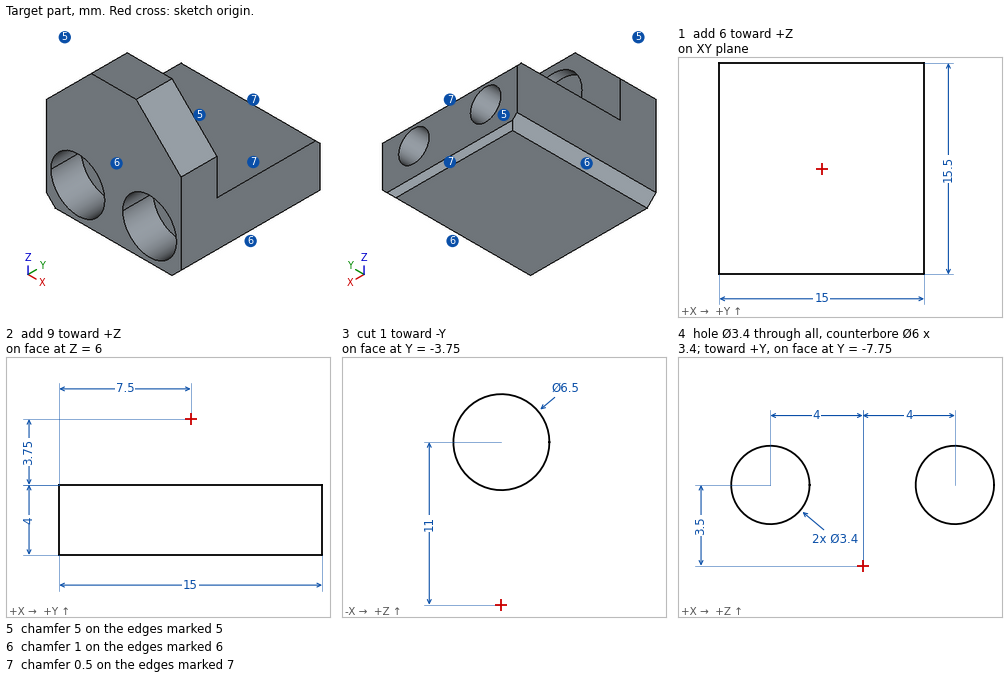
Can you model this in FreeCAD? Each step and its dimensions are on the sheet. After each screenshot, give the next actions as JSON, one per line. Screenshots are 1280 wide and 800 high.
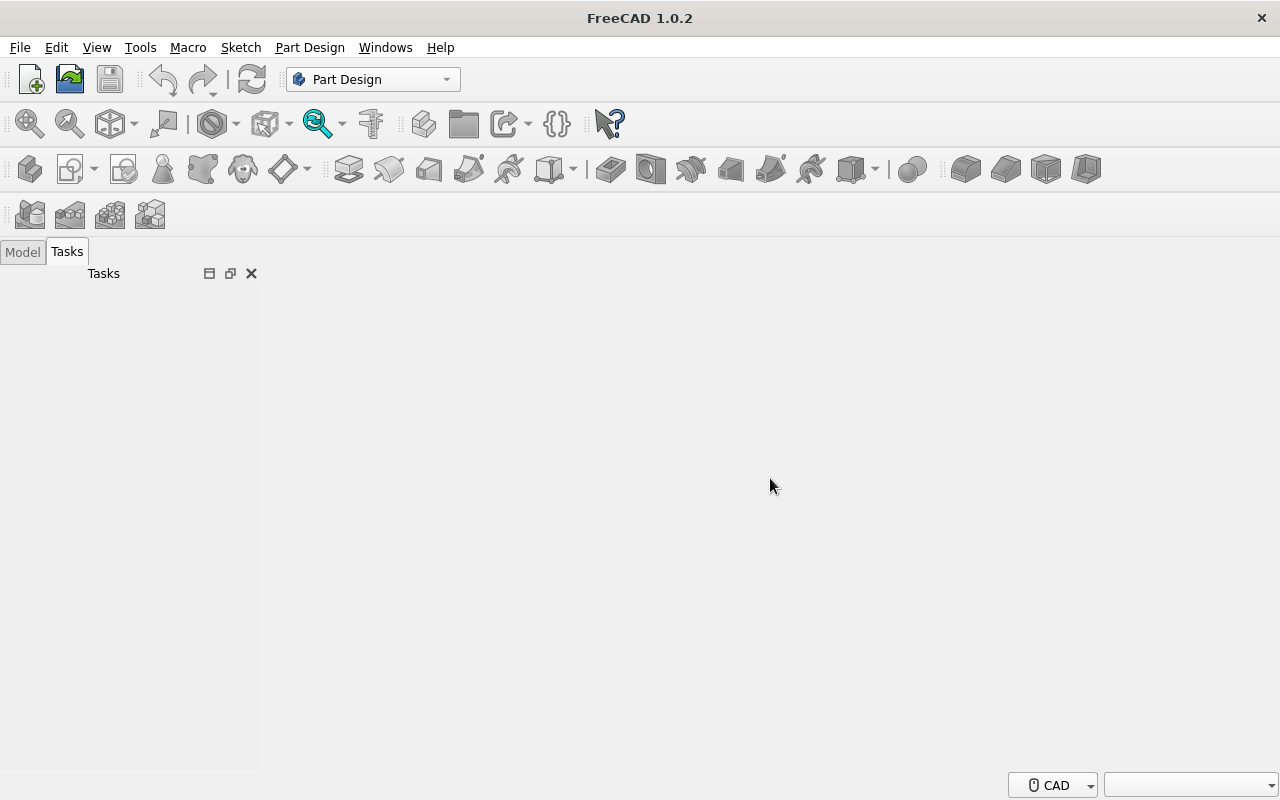
{"action": "left_click", "coordinate": [30, 80]}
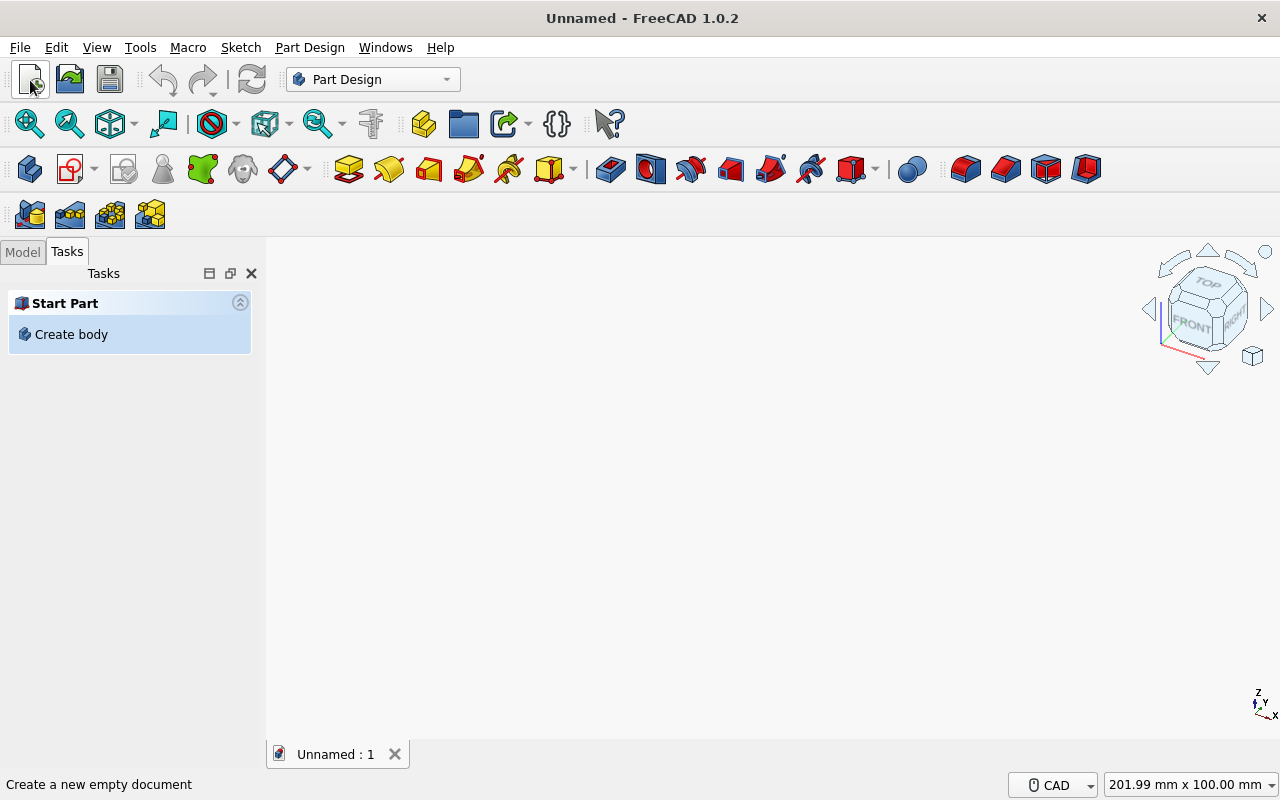
{"action": "left_click", "coordinate": [70, 170]}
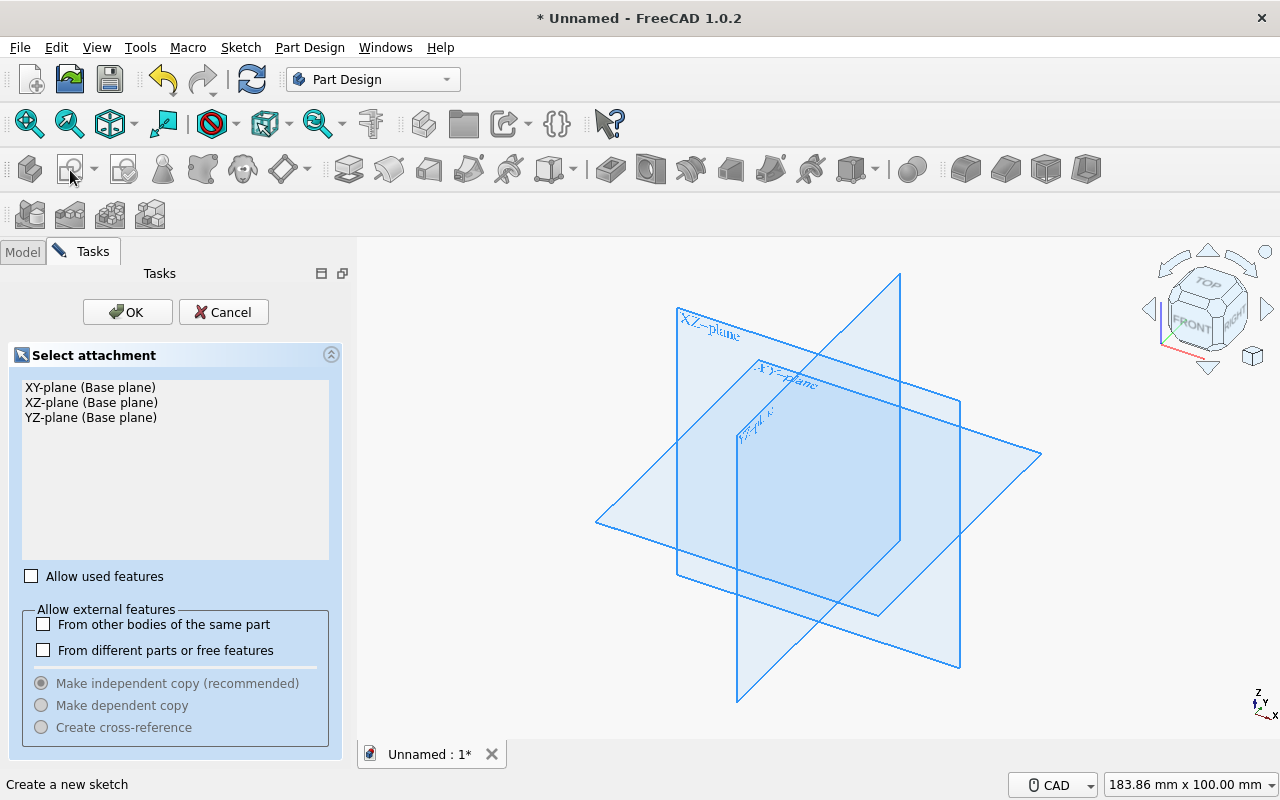
{"action": "left_click", "coordinate": [82, 388]}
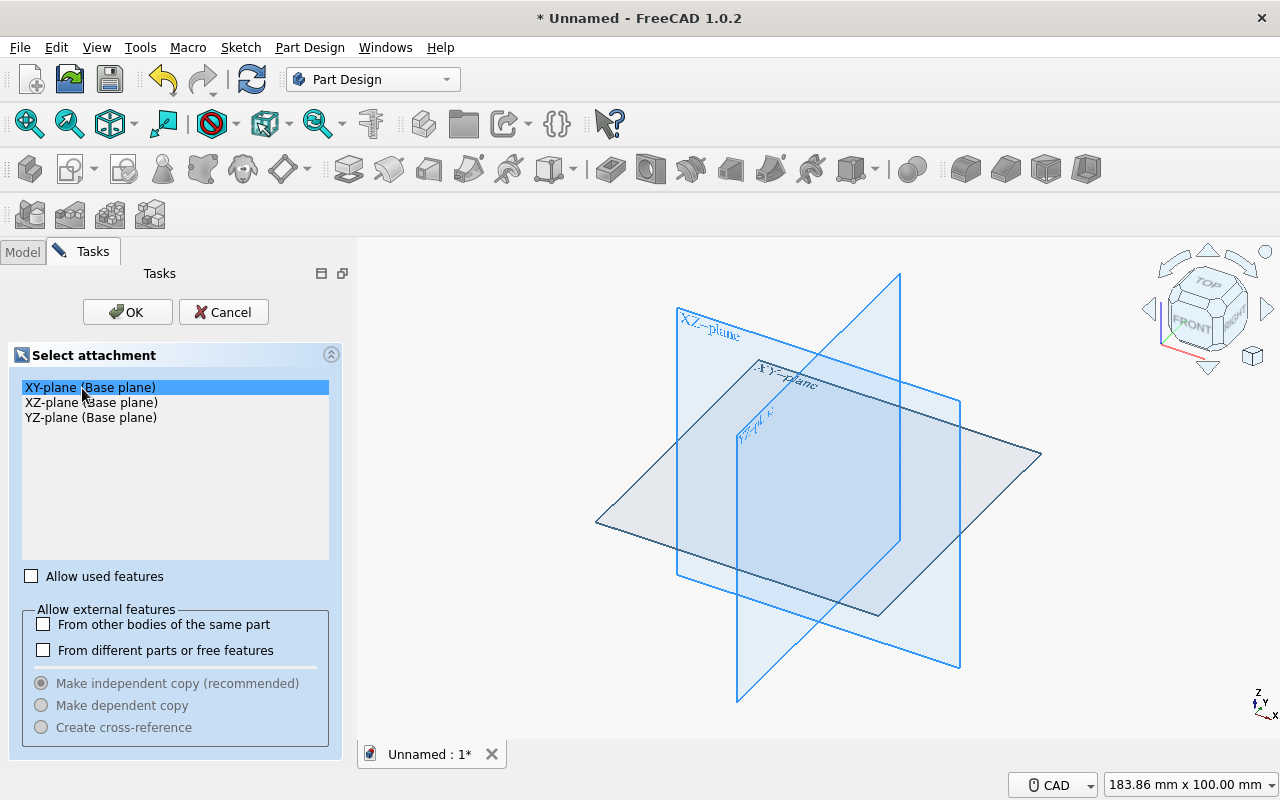
{"action": "left_click", "coordinate": [128, 312]}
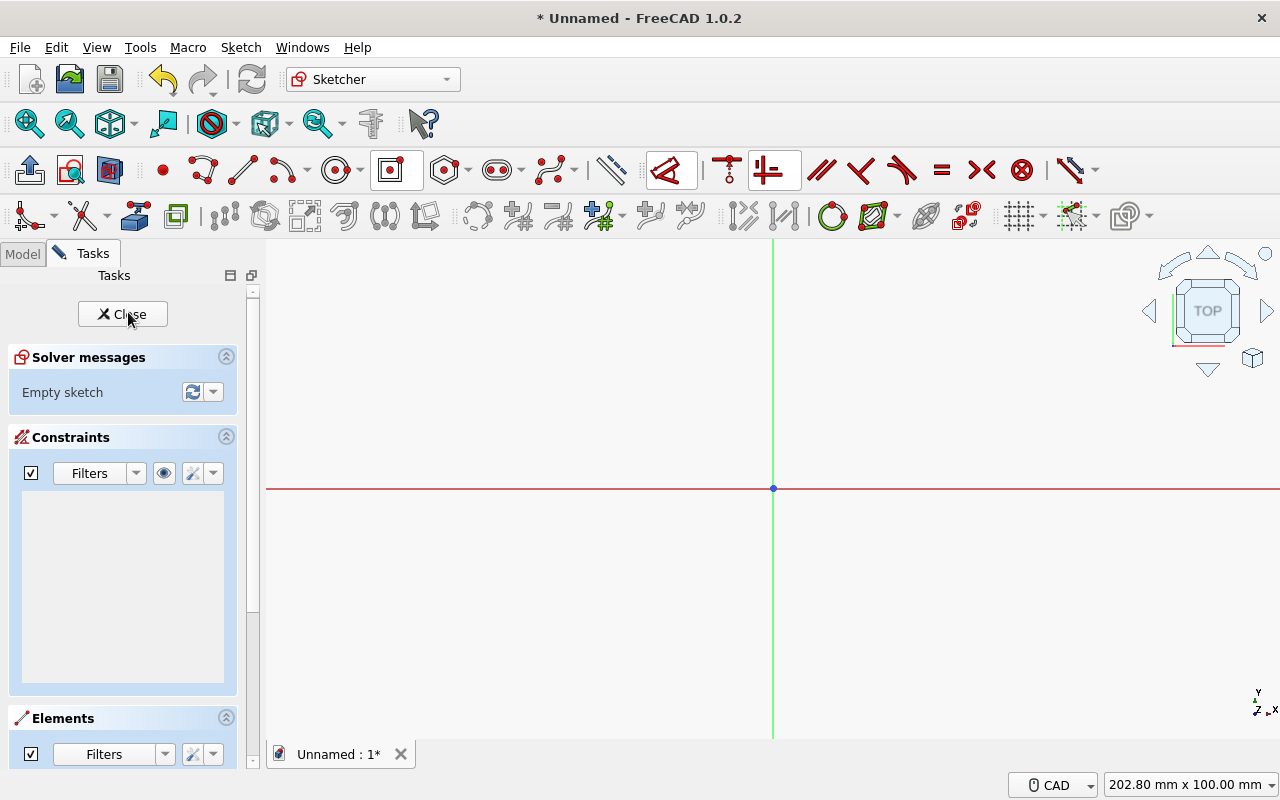
{"action": "scroll", "coordinate": [795, 489], "scroll_direction": "up", "scroll_amount": 7}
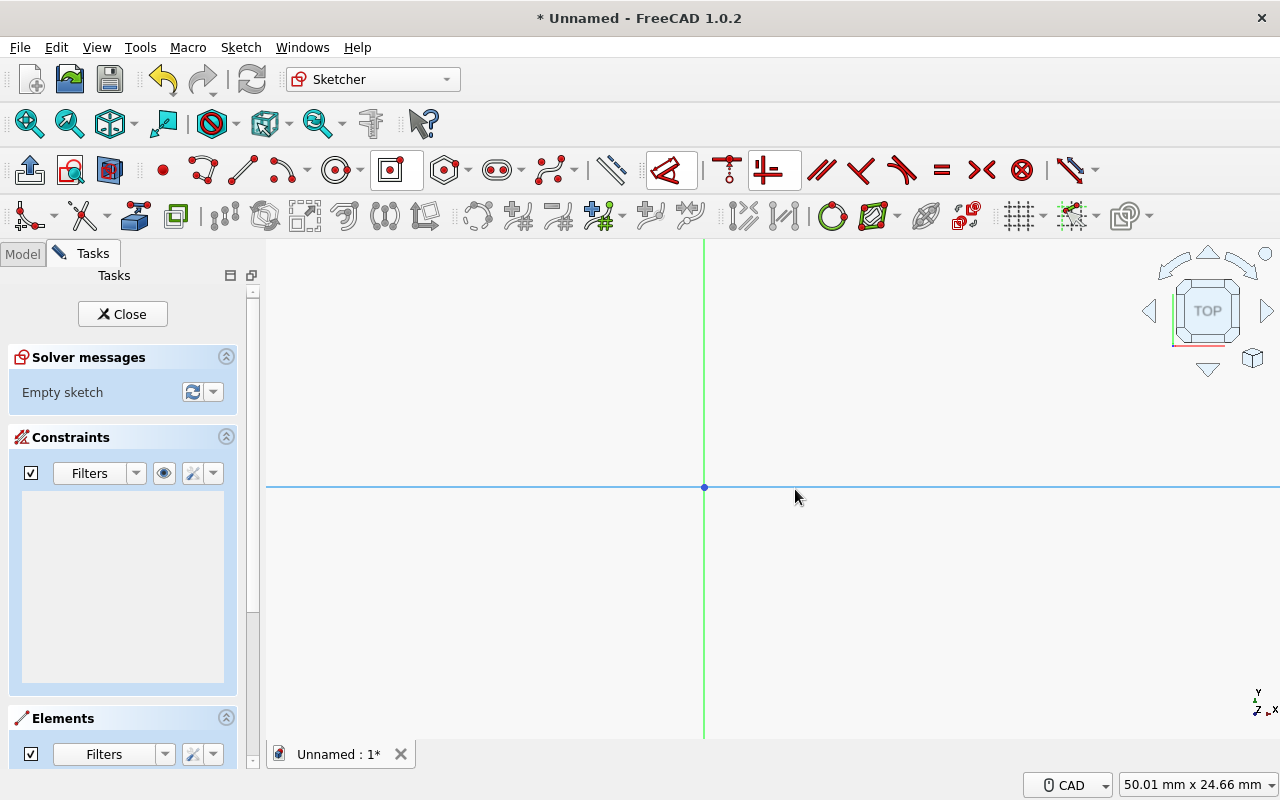
{"action": "key", "text": "g v"}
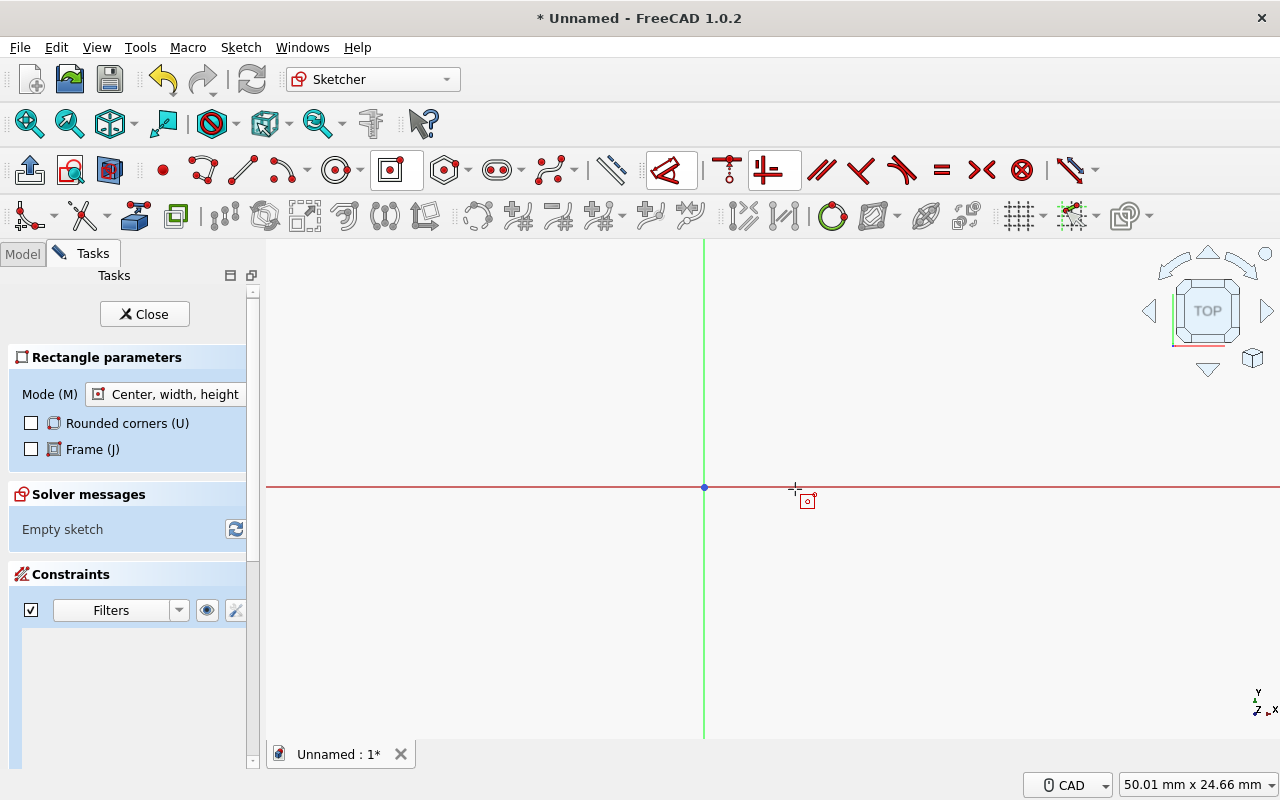
{"action": "left_click", "coordinate": [704, 487]}
{"action": "left_click", "coordinate": [856, 330]}
{"action": "key", "text": "Escape"}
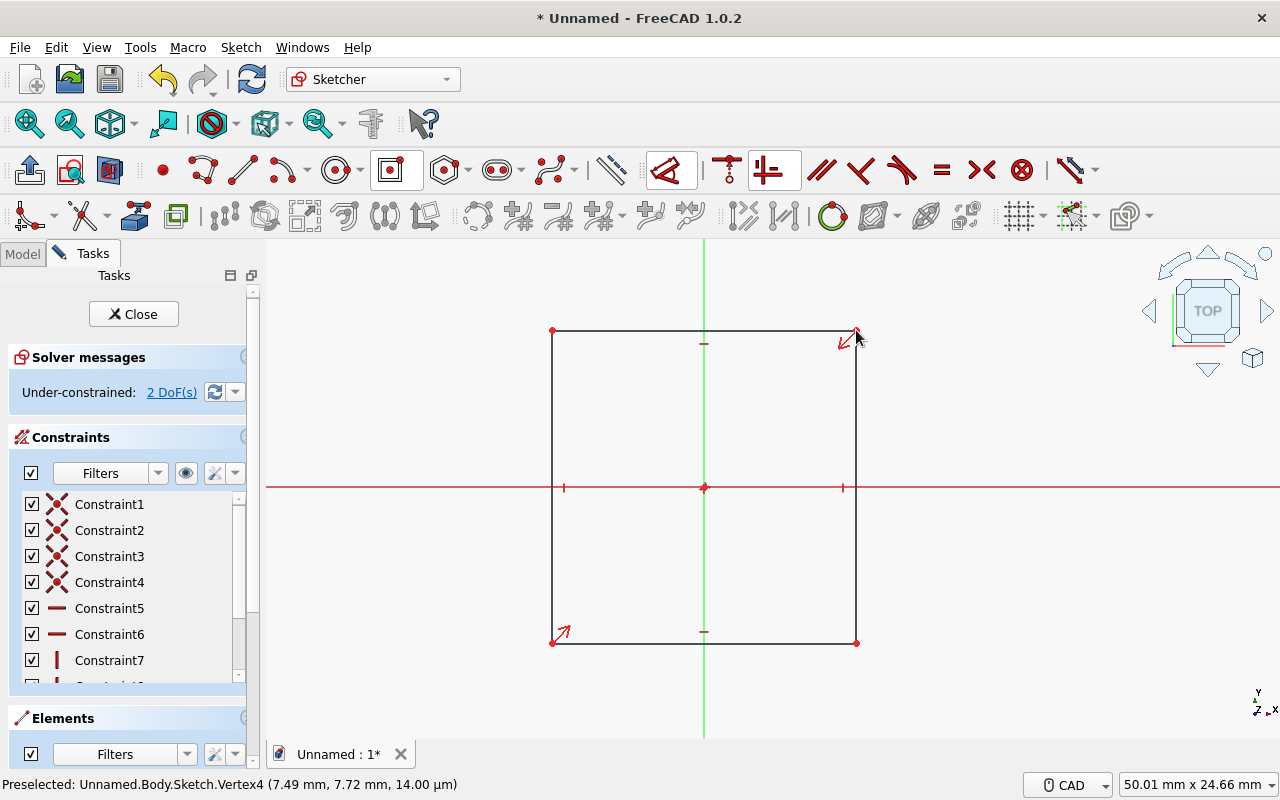
{"action": "key", "text": "d"}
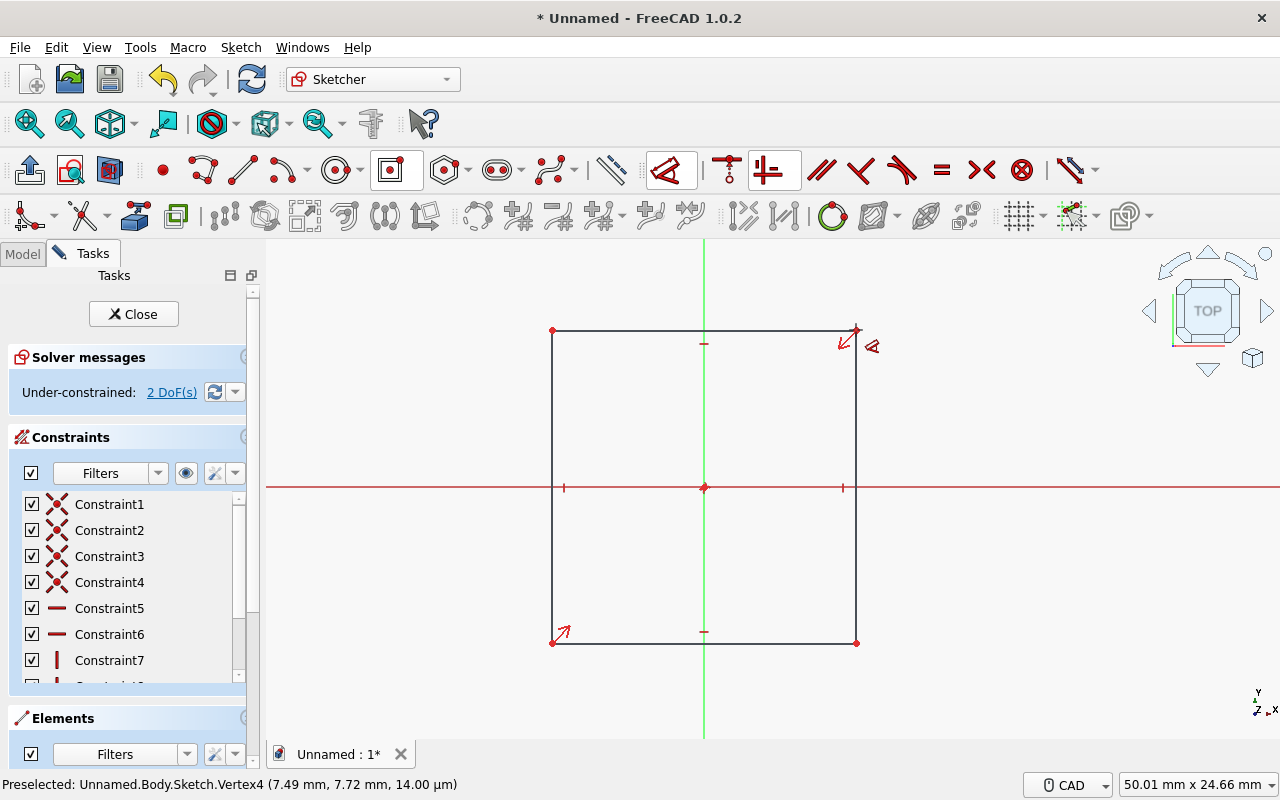
{"action": "left_click", "coordinate": [643, 644]}
{"action": "left_click", "coordinate": [634, 678]}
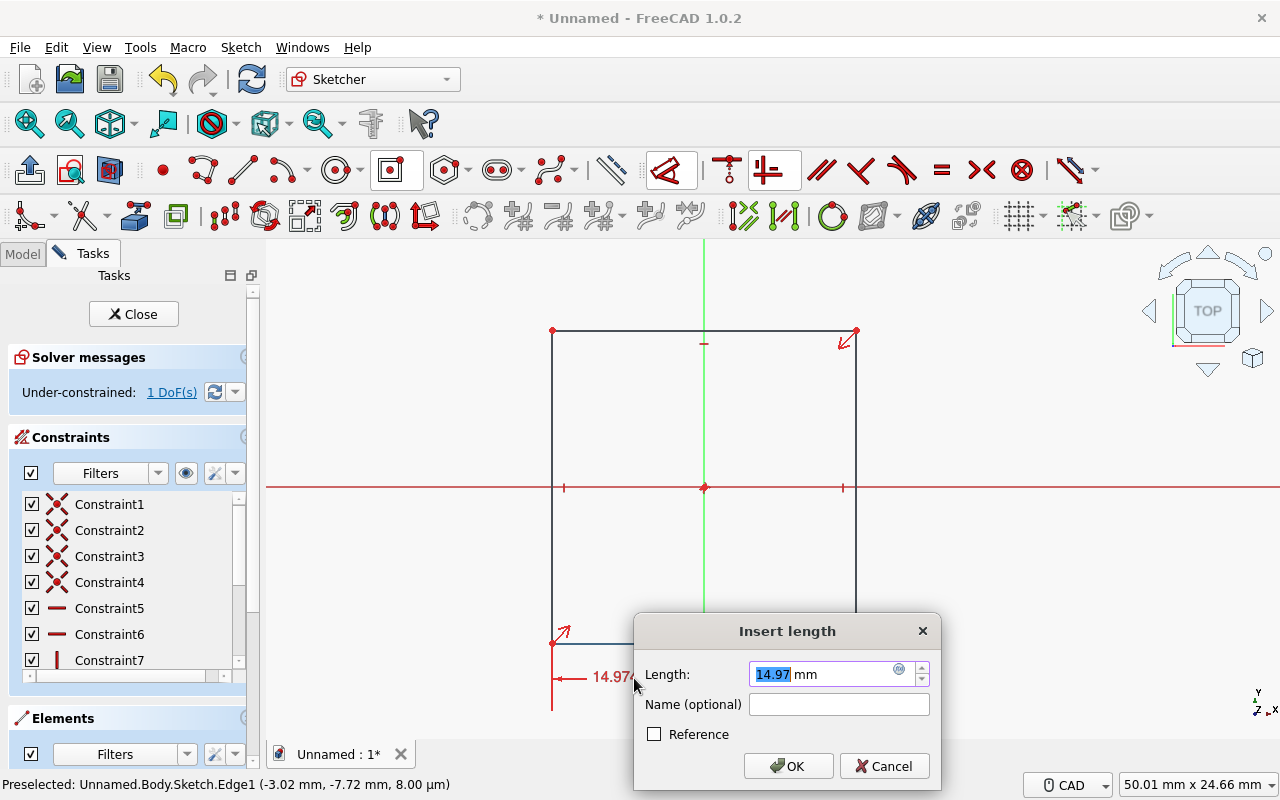
{"action": "type", "text": "15"}
{"action": "key", "text": "Return"}